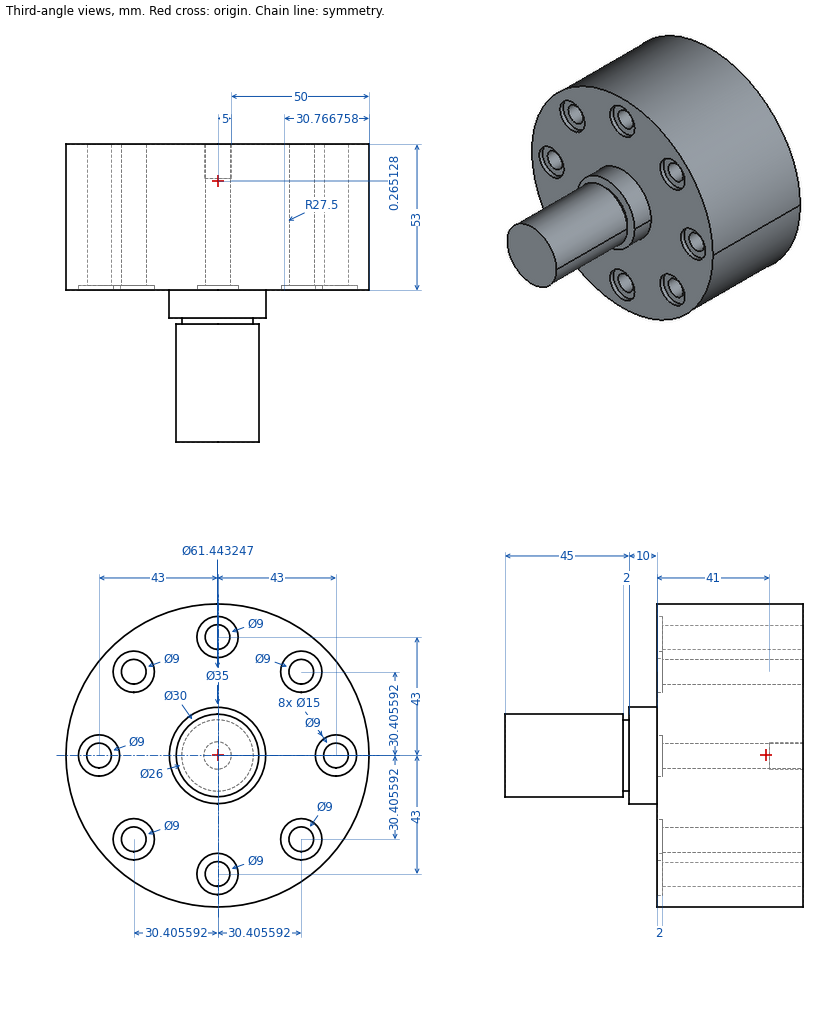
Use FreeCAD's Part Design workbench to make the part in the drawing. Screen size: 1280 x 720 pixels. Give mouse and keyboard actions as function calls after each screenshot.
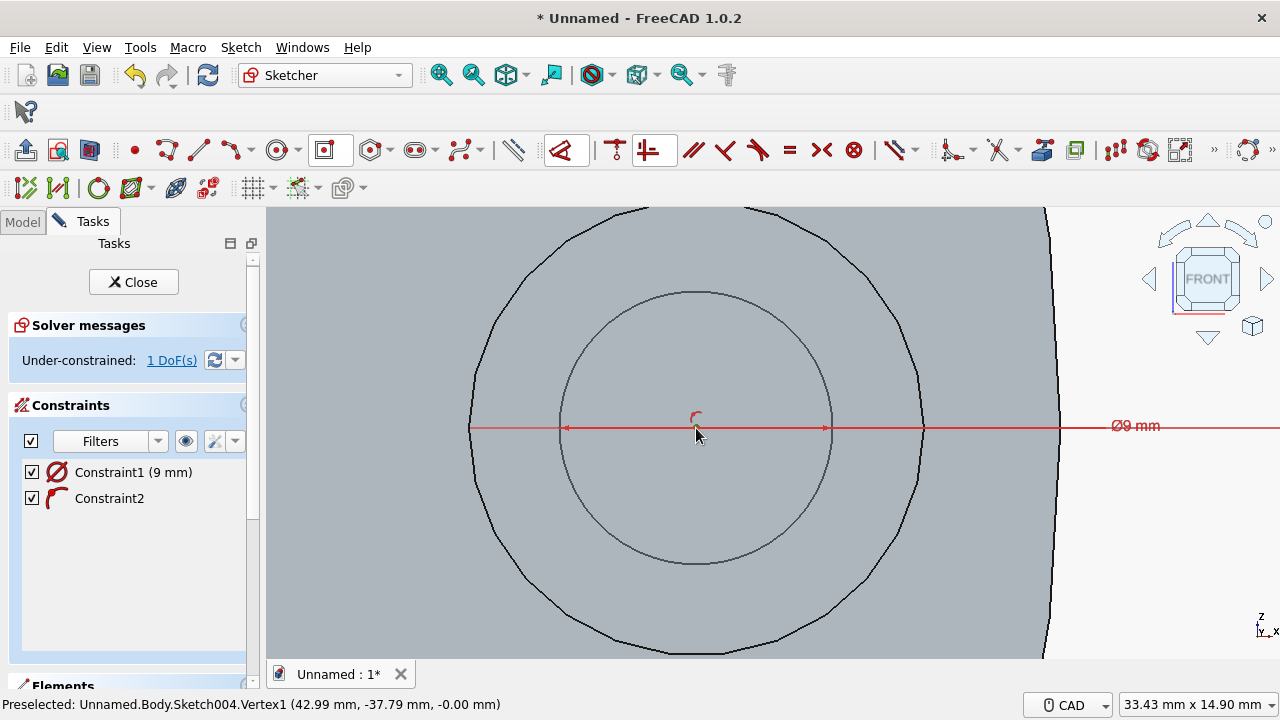
click(584, 150)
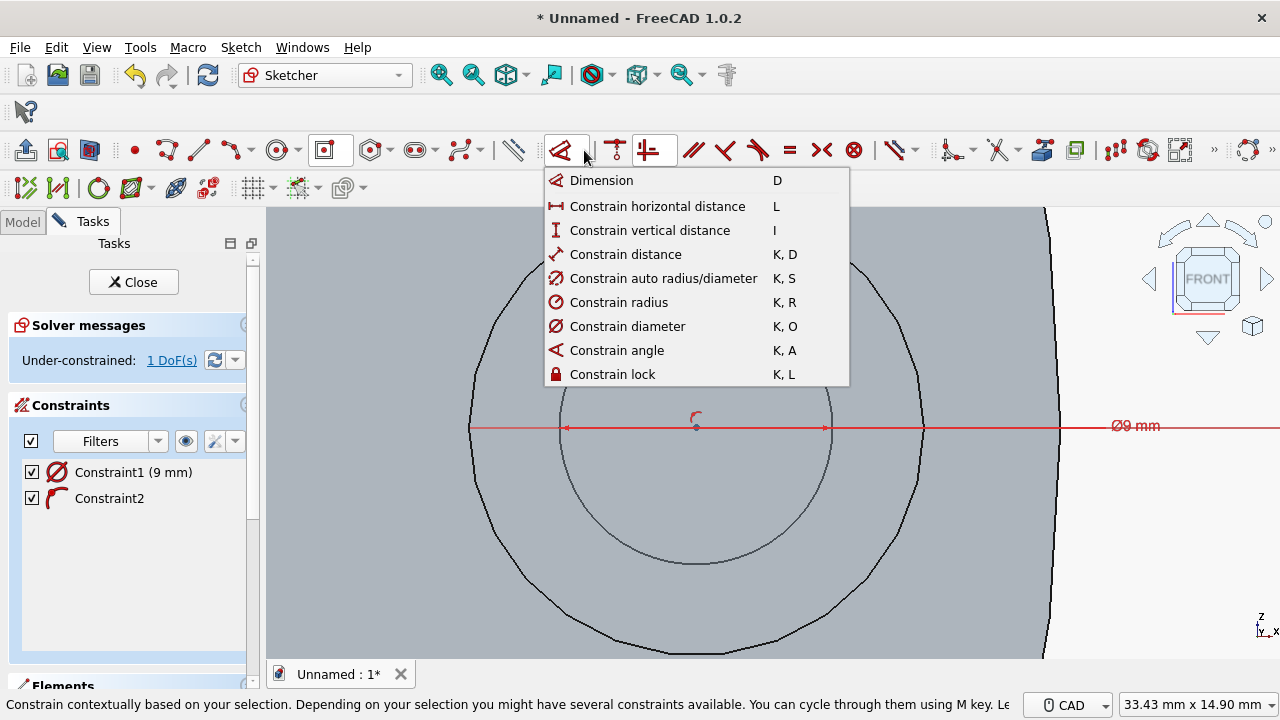
click(697, 206)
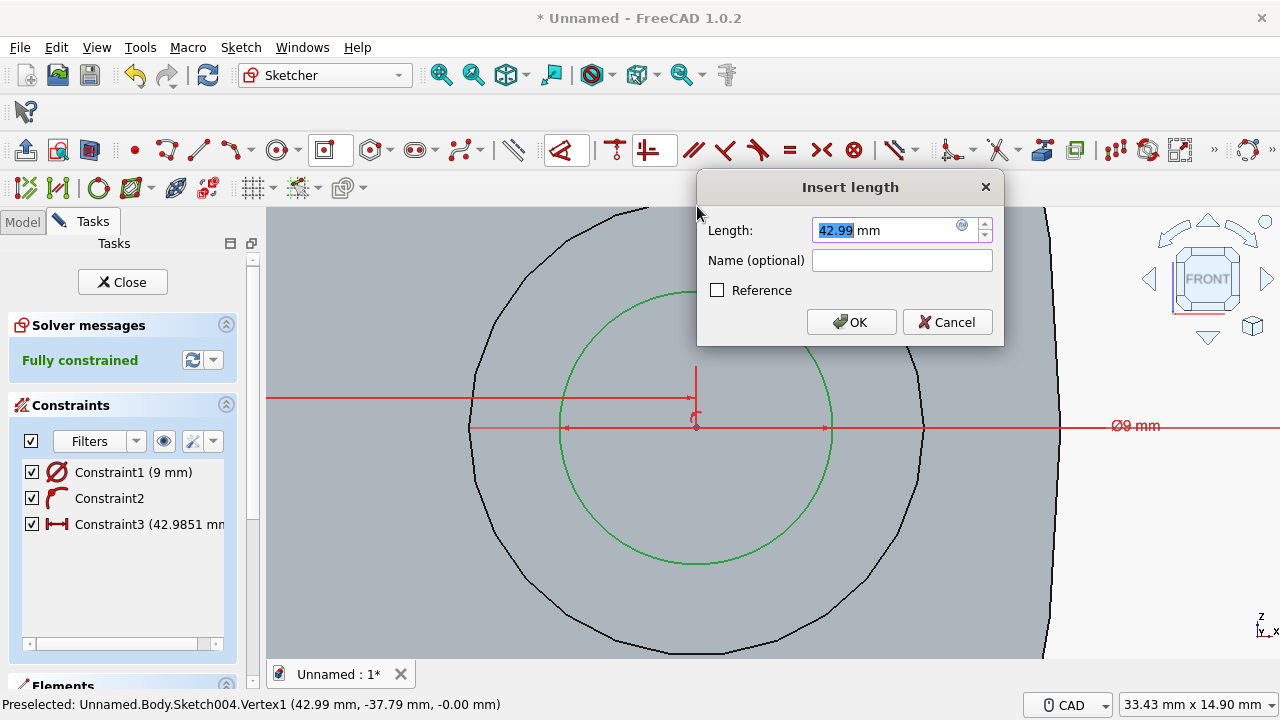
text(43)
key(Return)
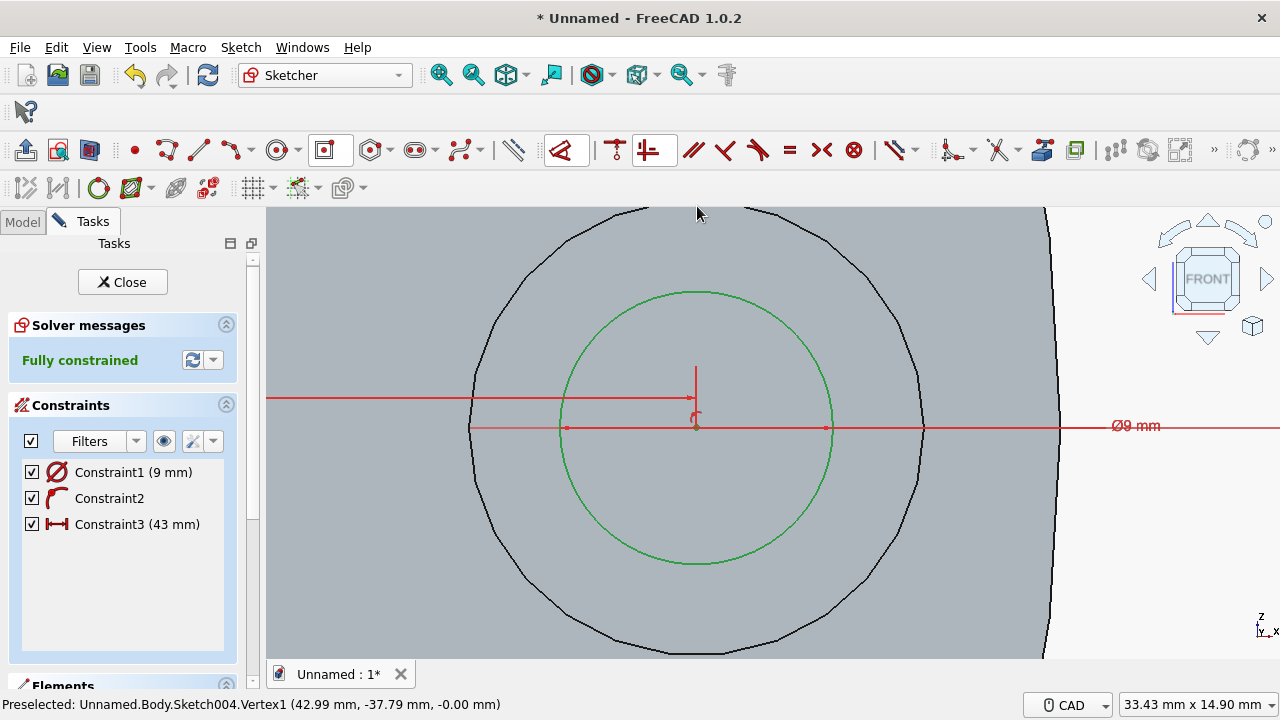
click(123, 282)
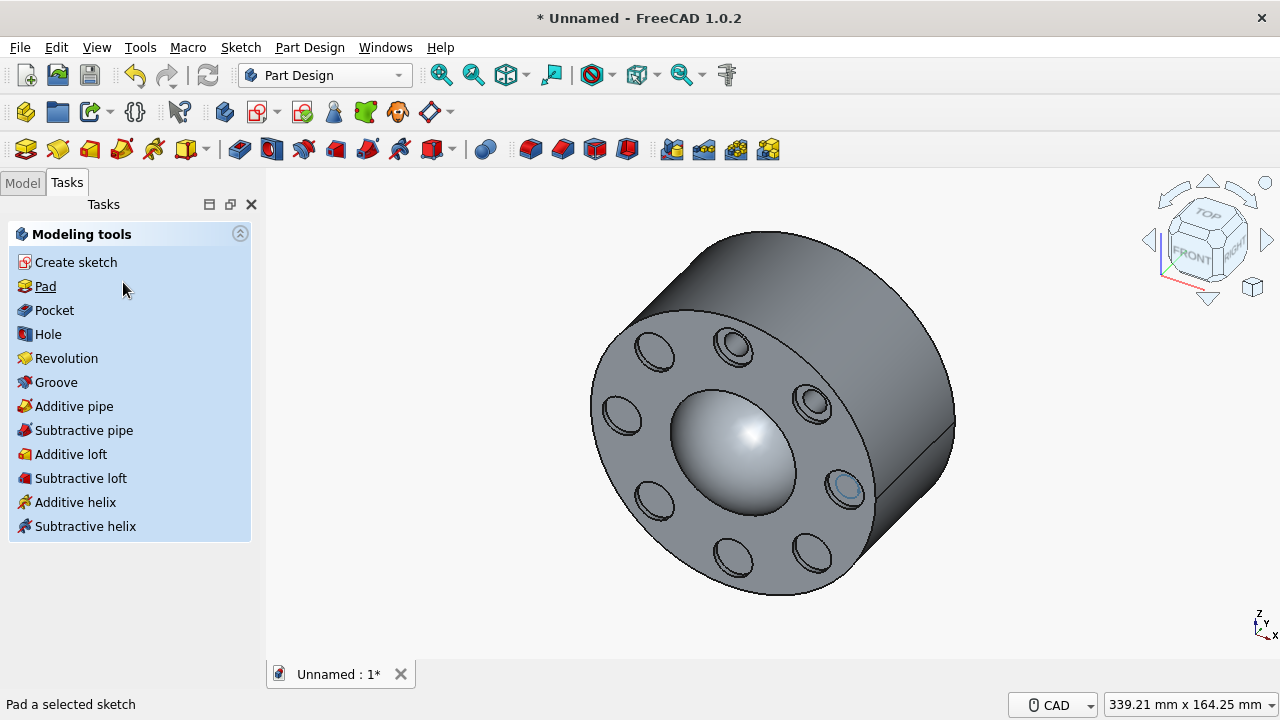
click(240, 150)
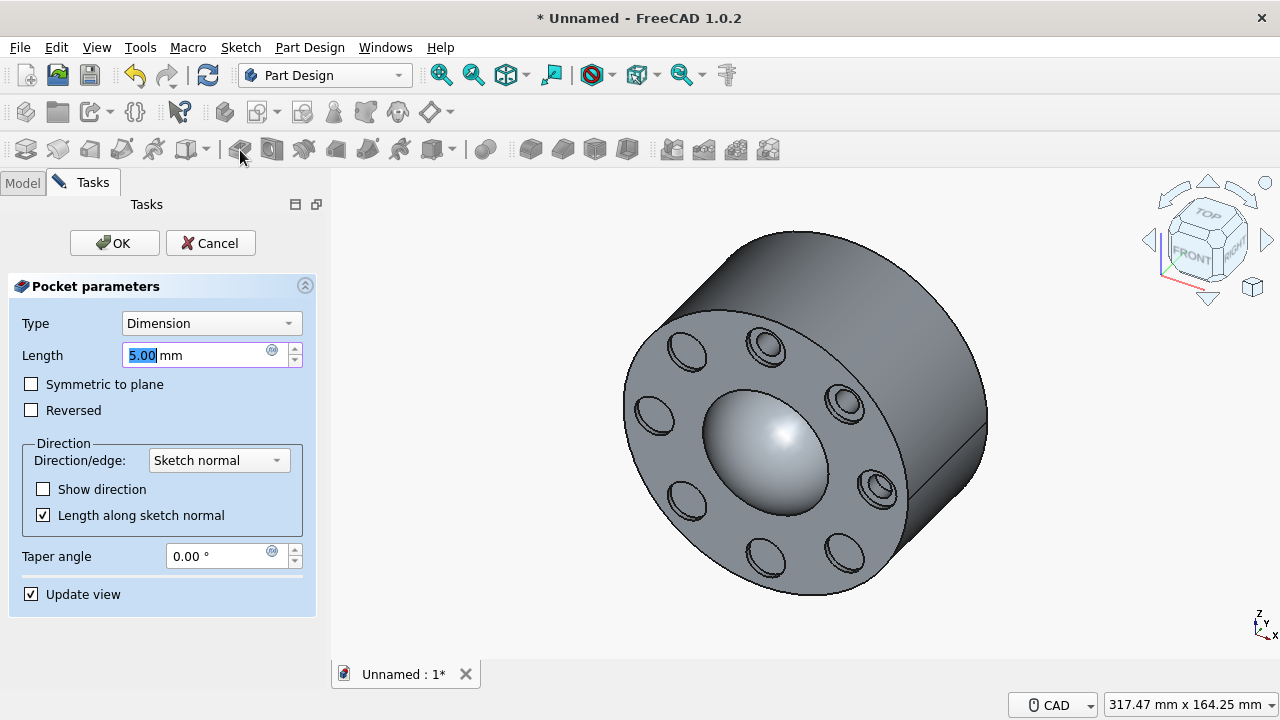
click(212, 324)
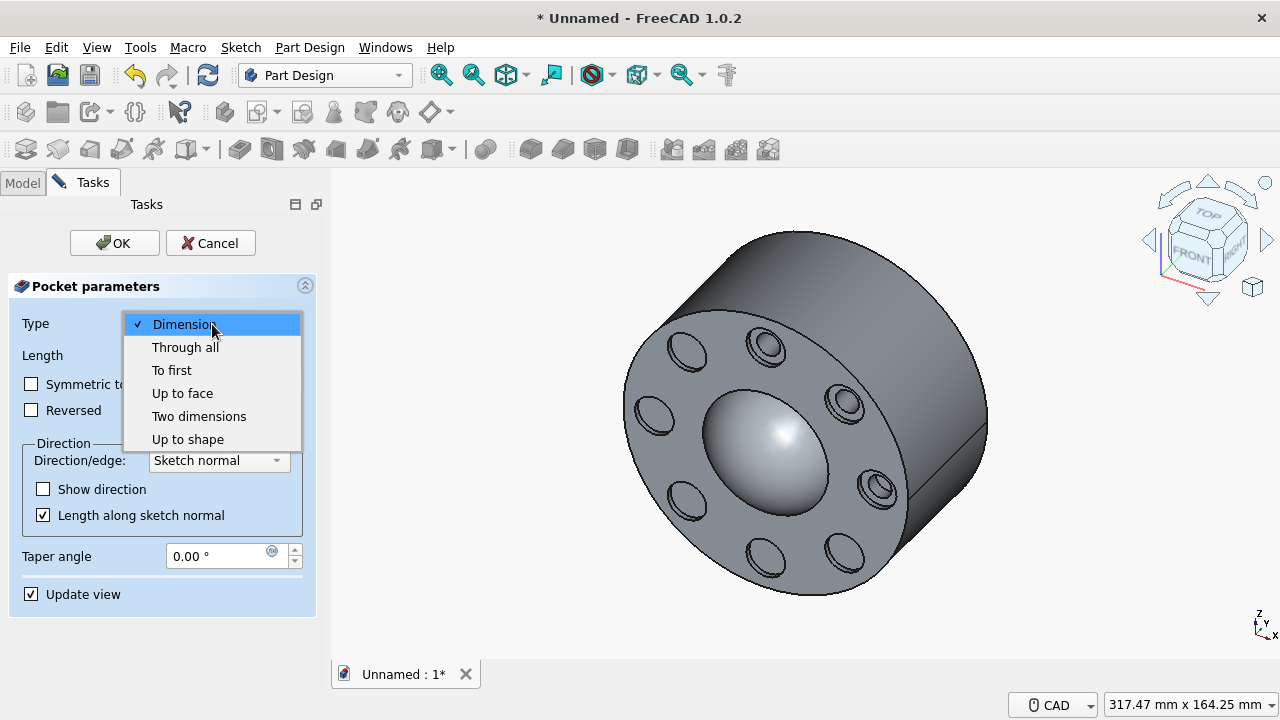
click(212, 370)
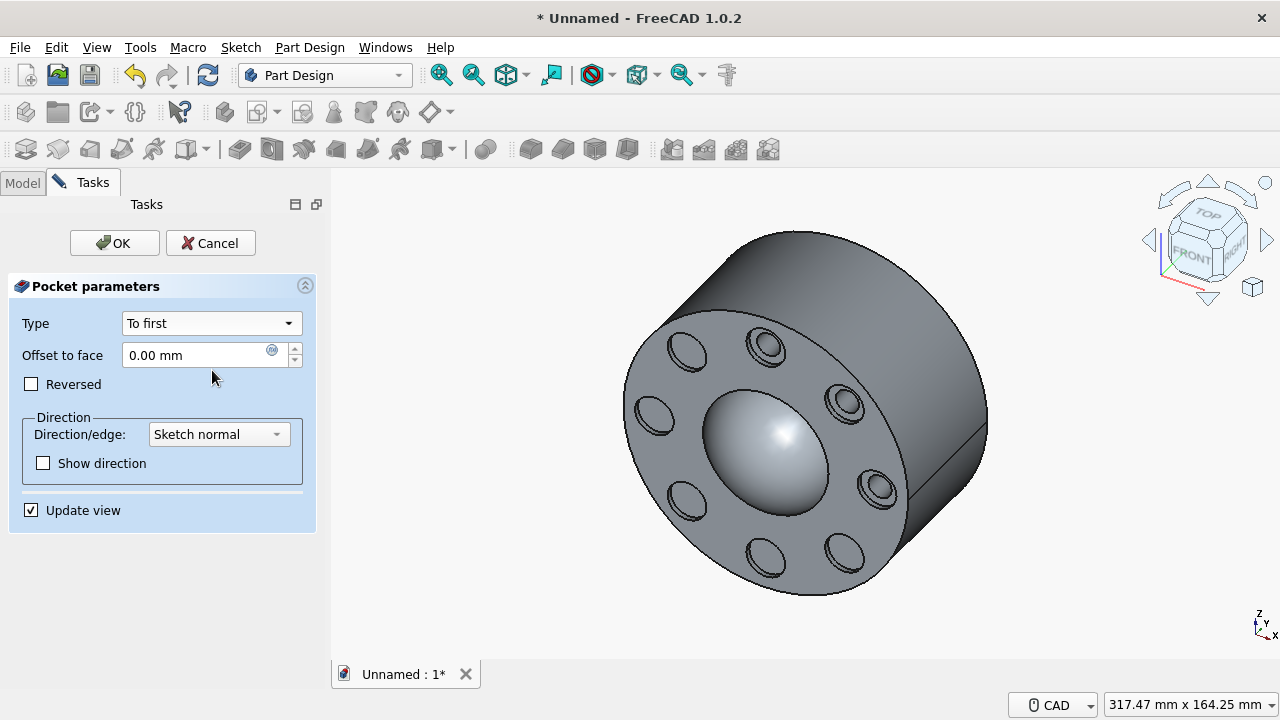
click(115, 243)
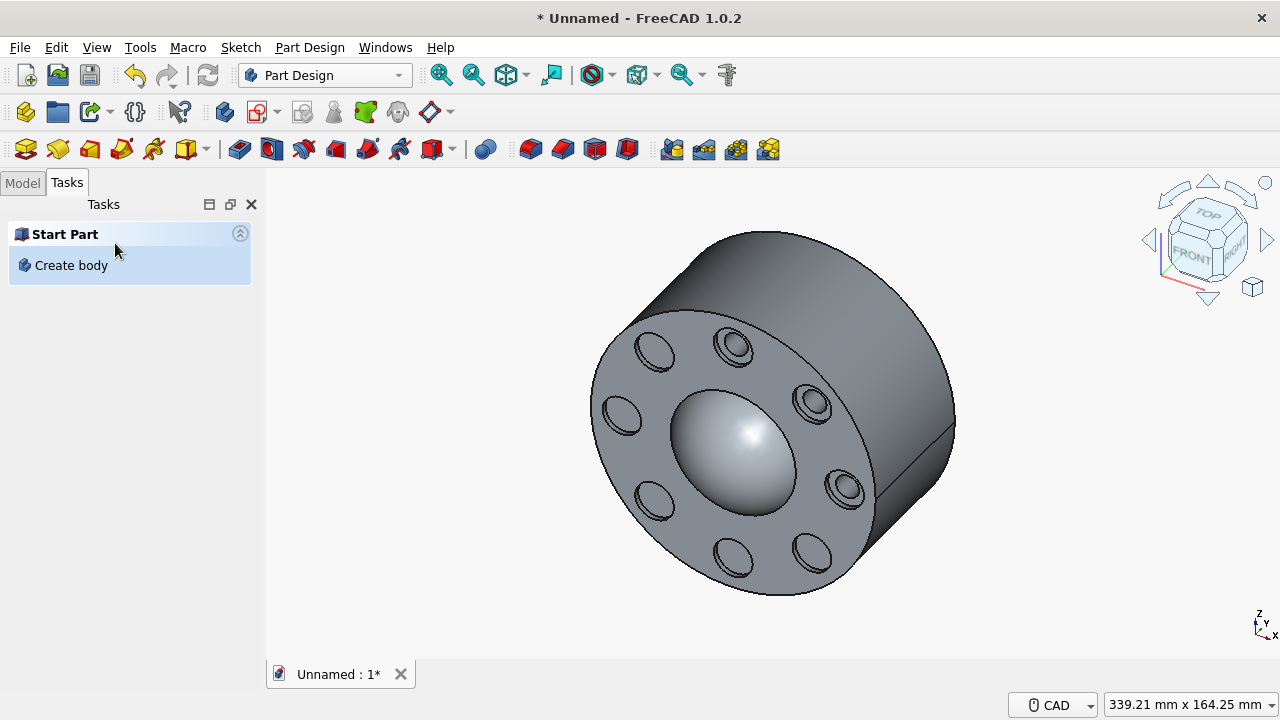
click(658, 348)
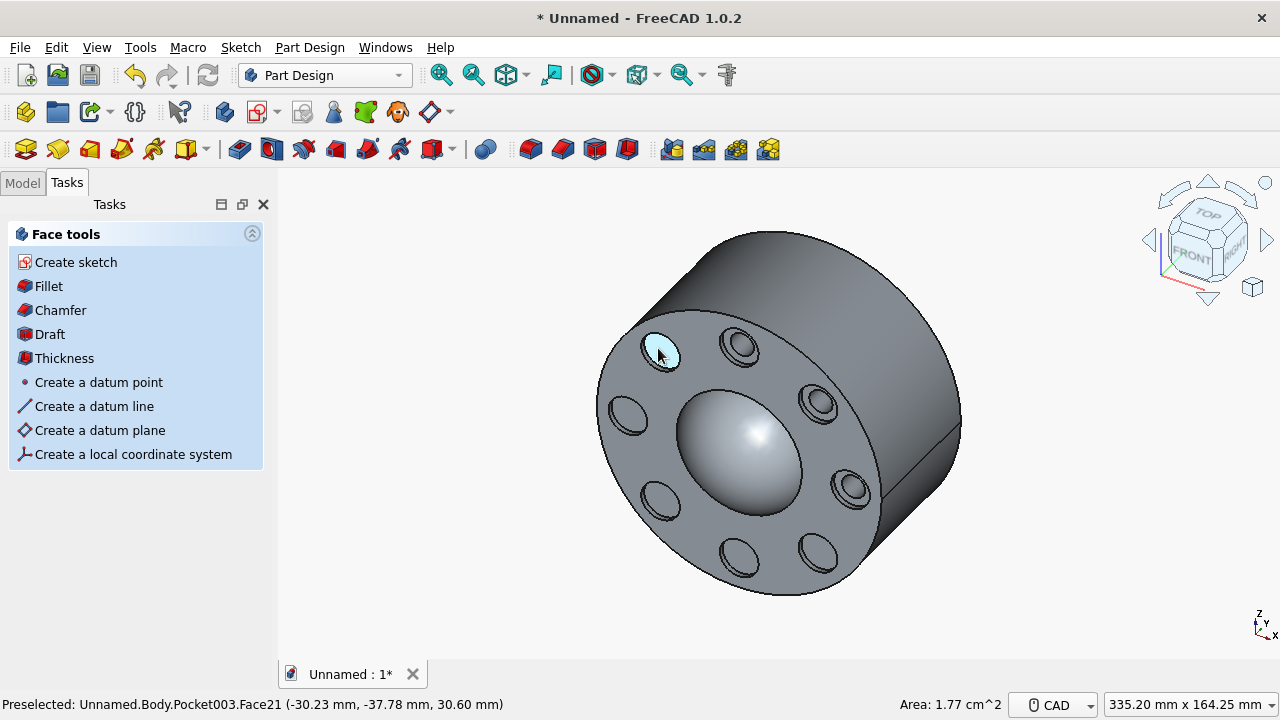
click(258, 112)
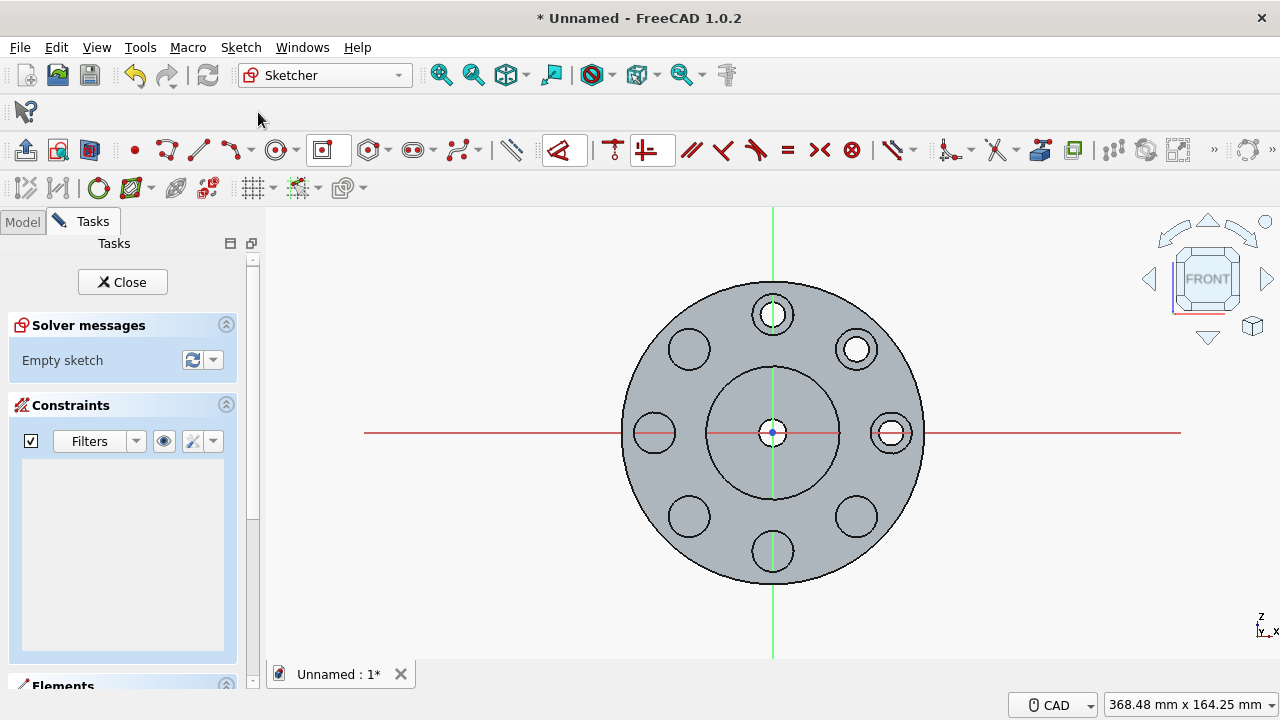
click(90, 150)